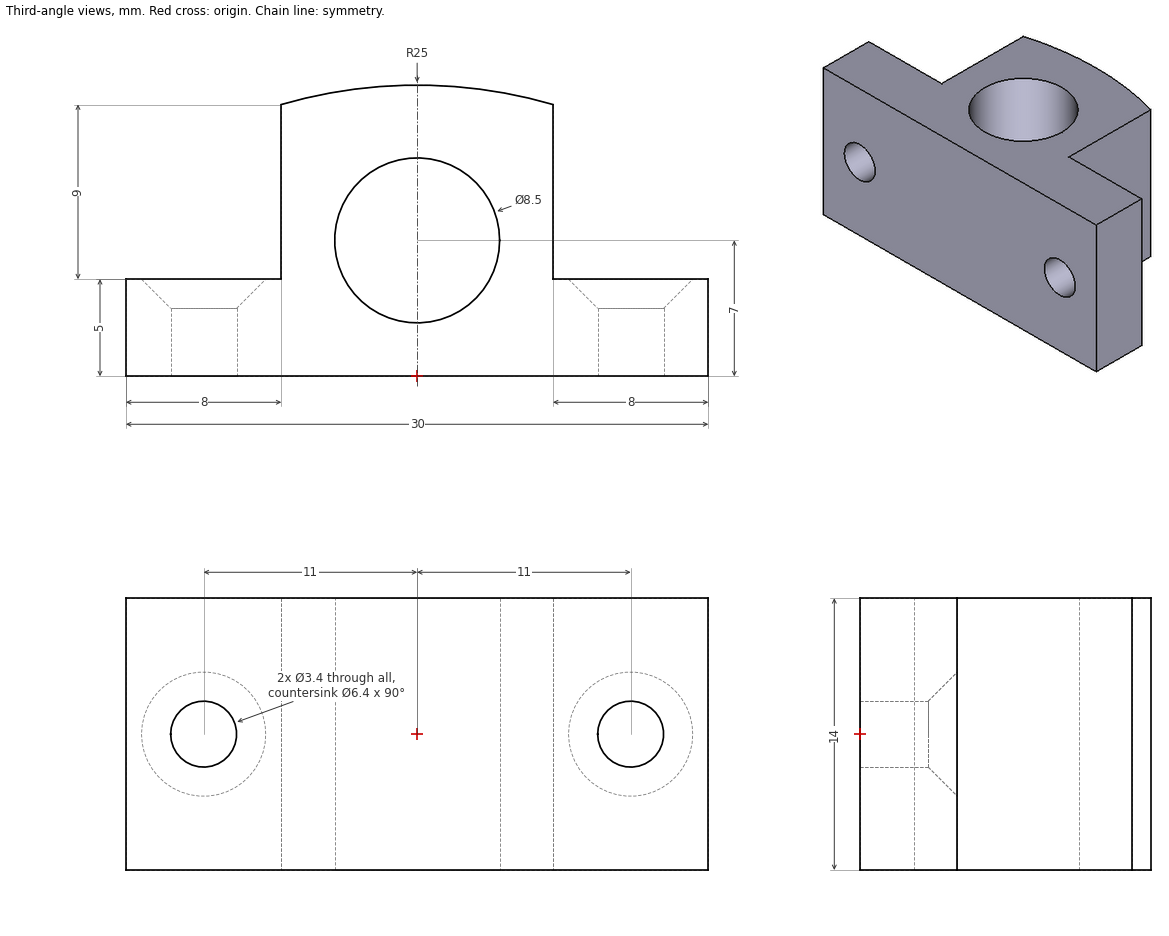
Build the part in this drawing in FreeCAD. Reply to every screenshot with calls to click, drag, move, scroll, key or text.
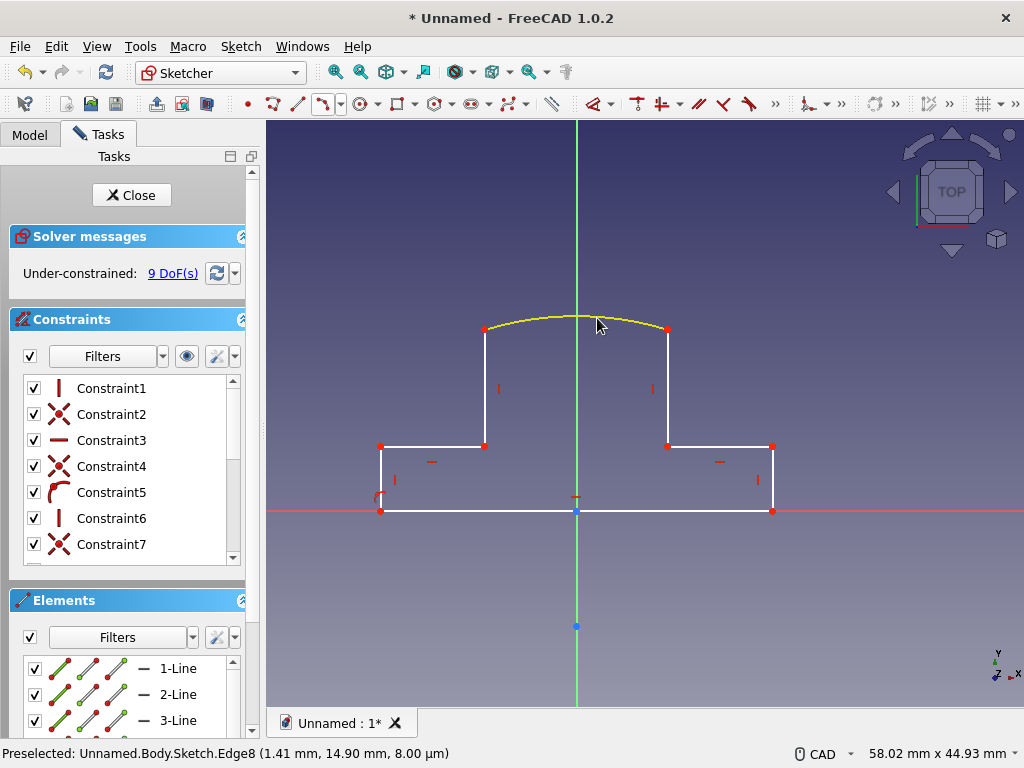
click(576, 627)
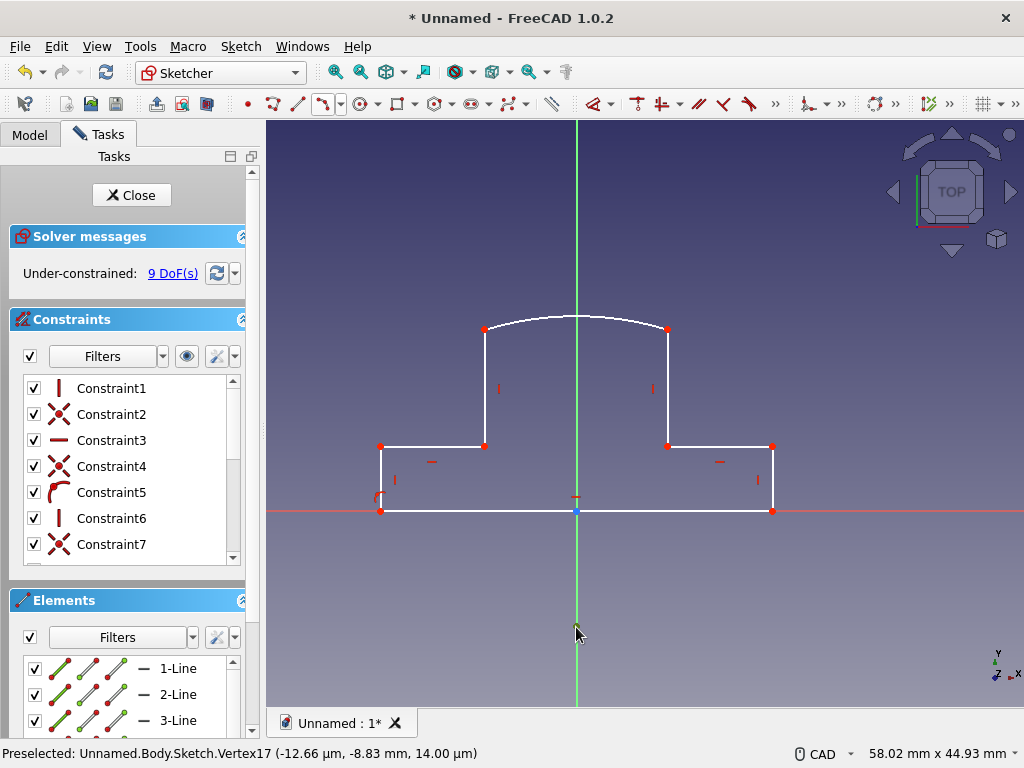
click(577, 641)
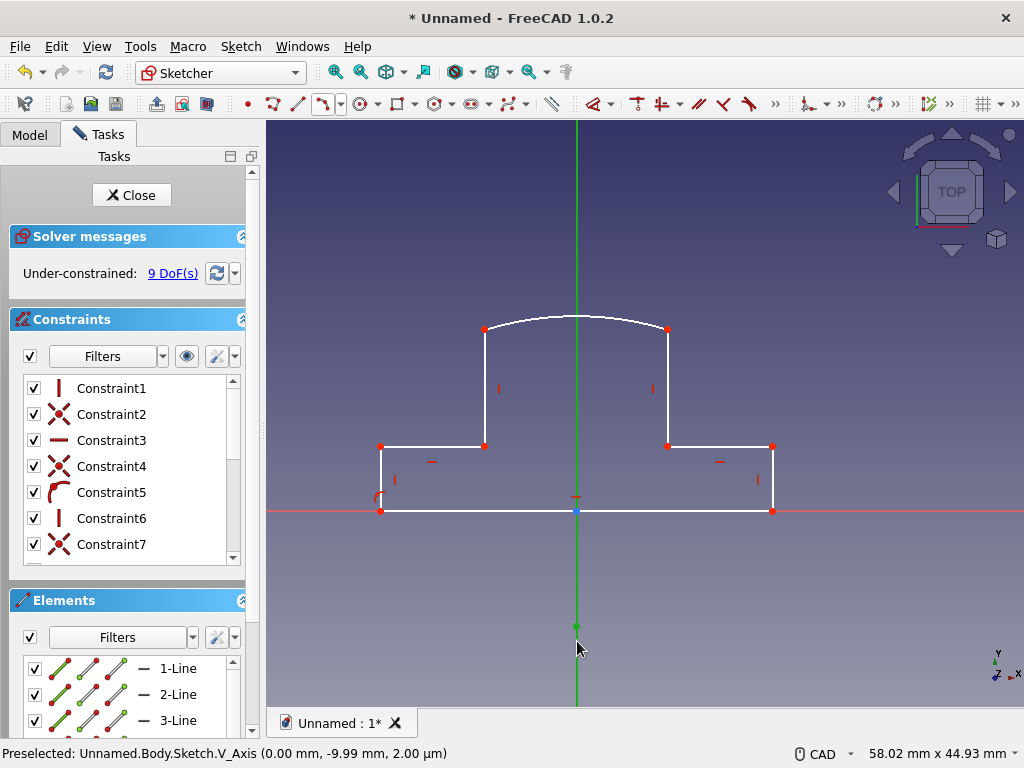
click(637, 104)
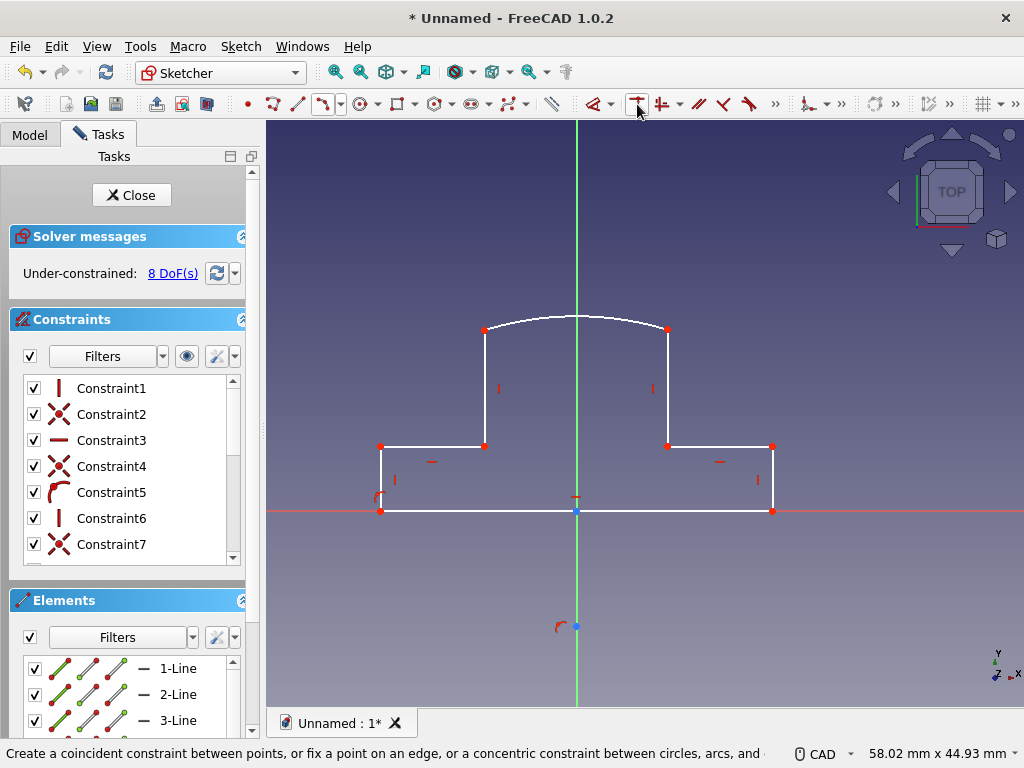
click(381, 447)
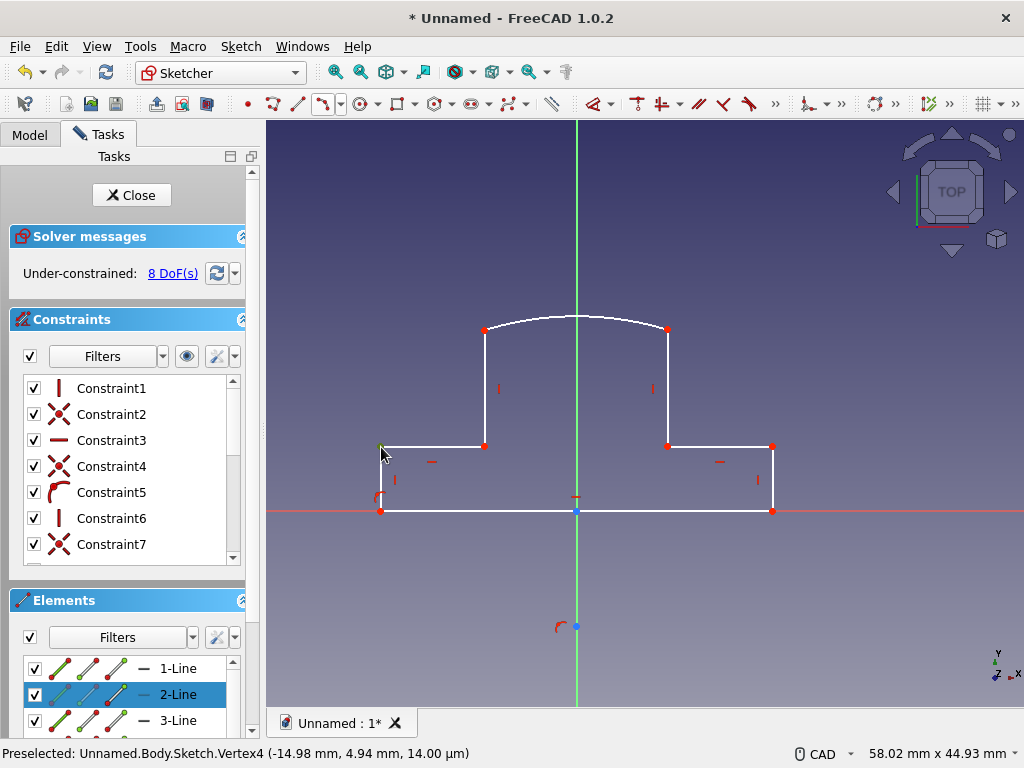
click(773, 447)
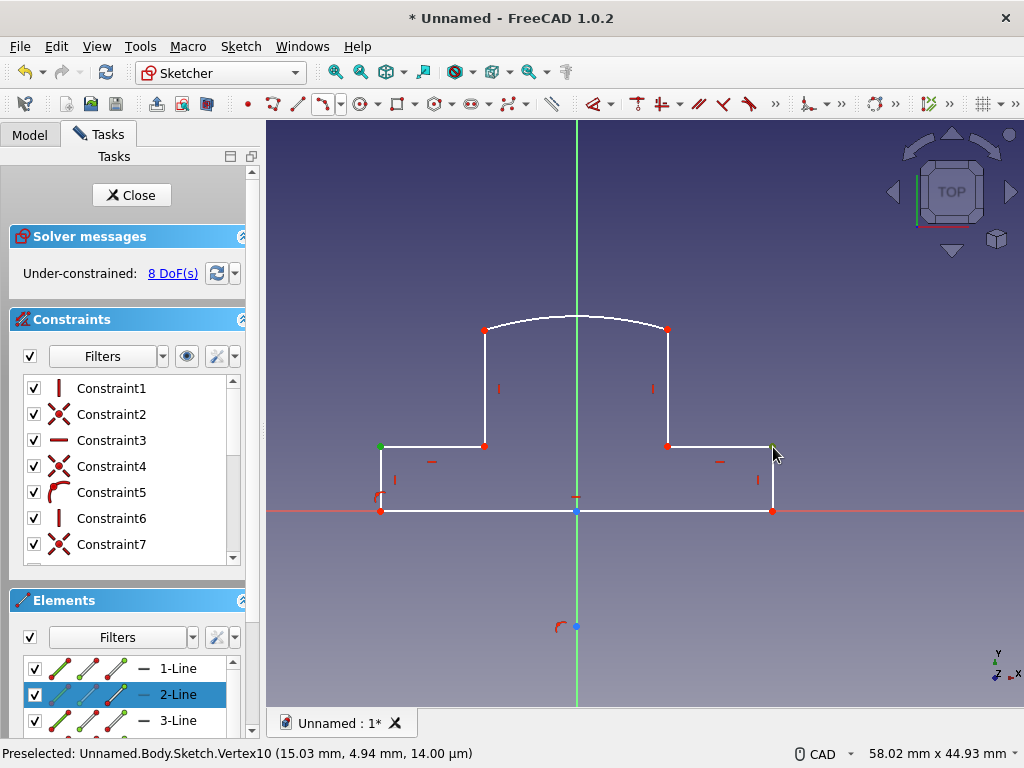
click(577, 641)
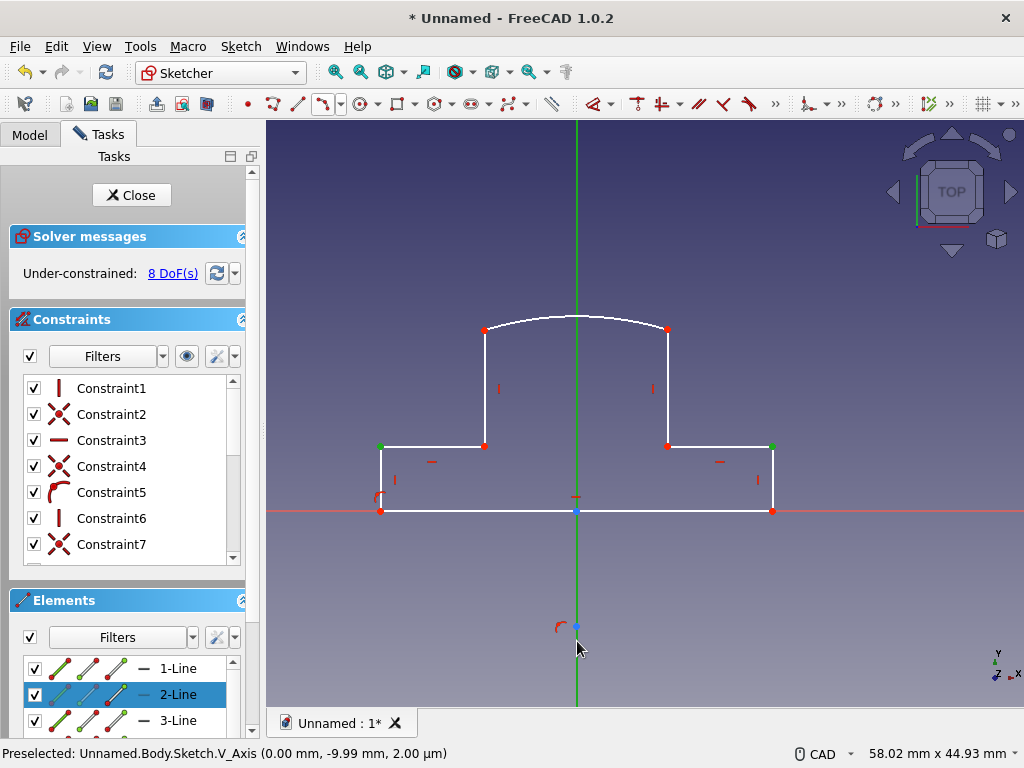
key(s)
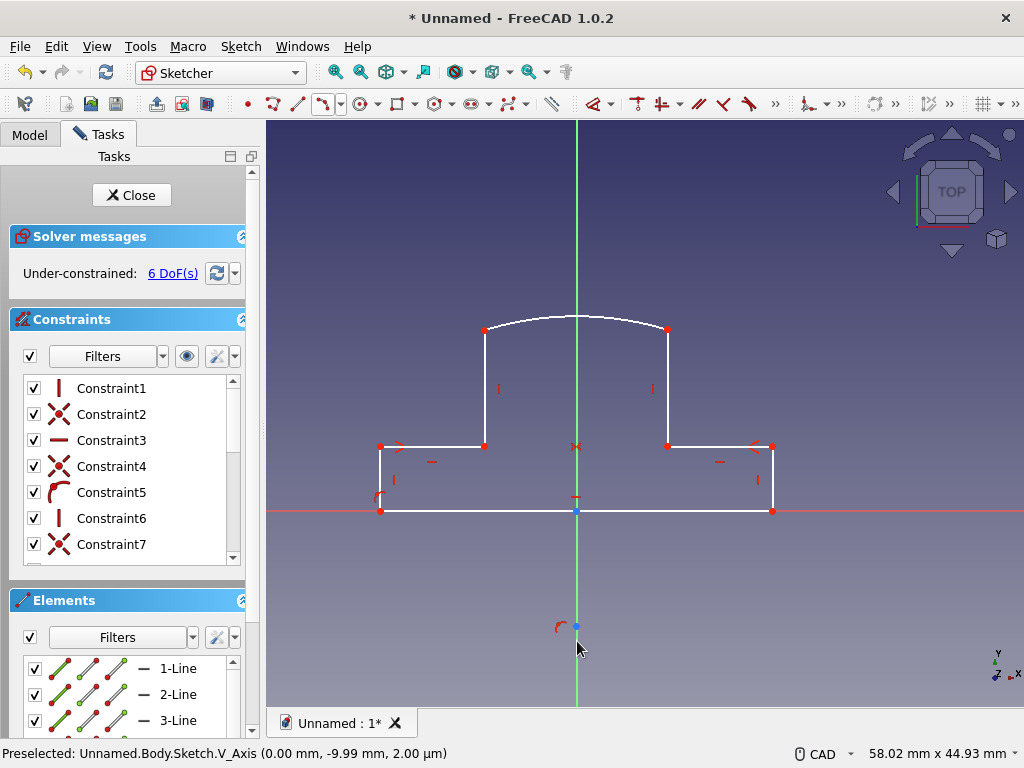
click(592, 104)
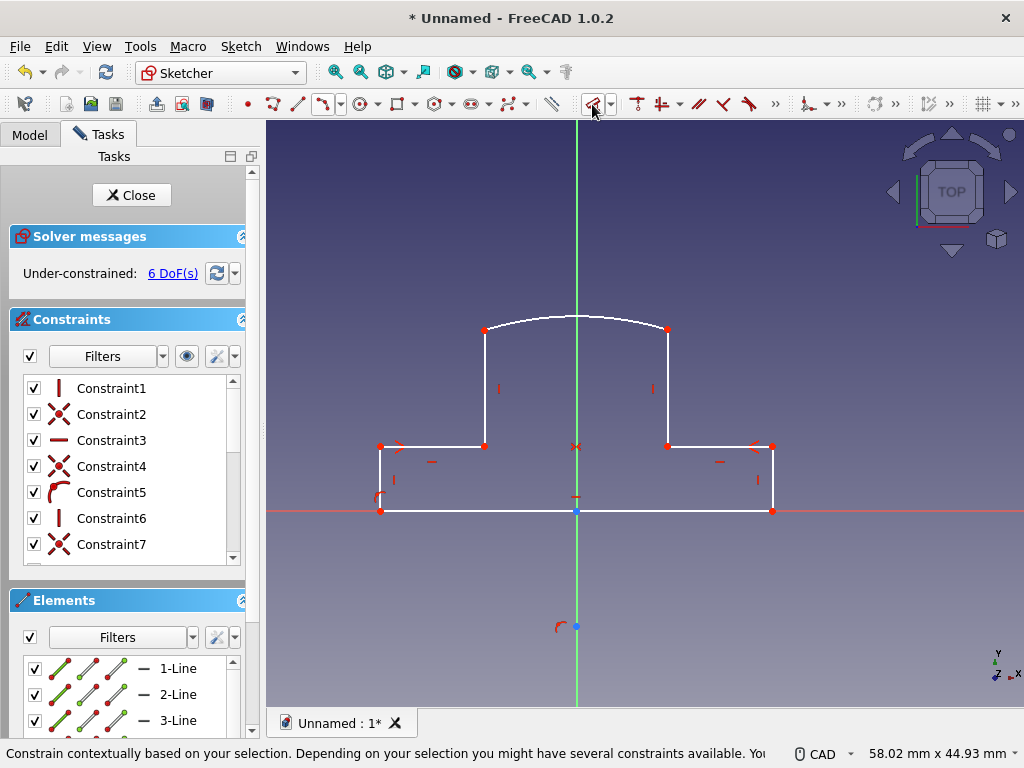
click(614, 318)
click(618, 286)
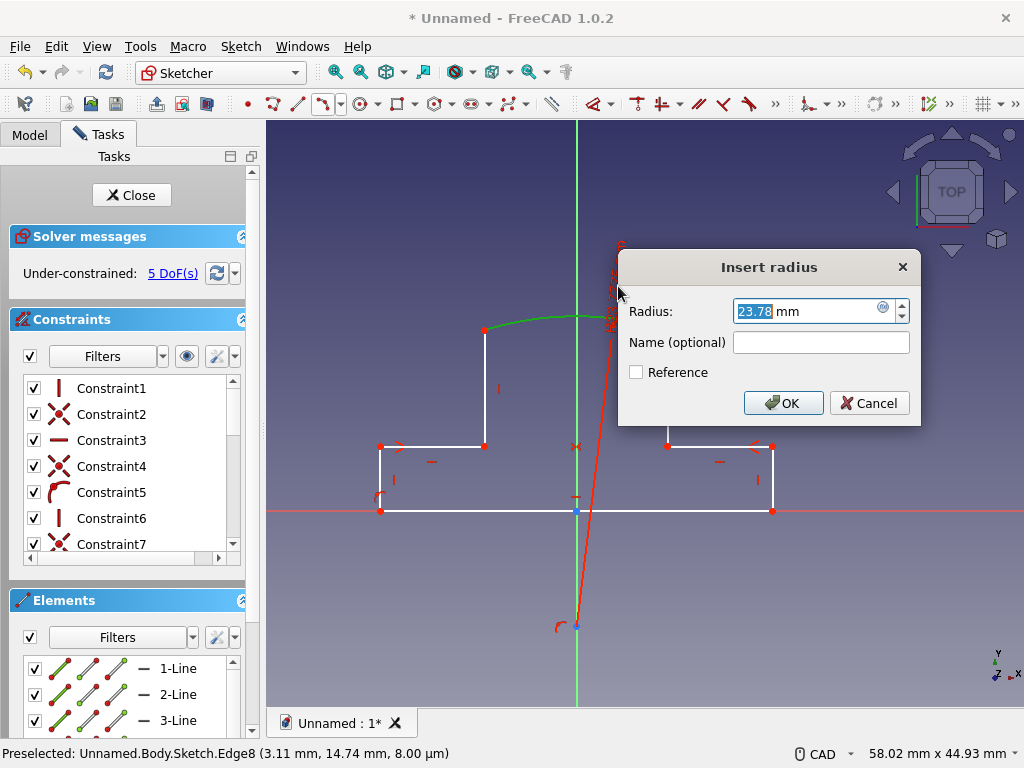
text(25)
key(Return)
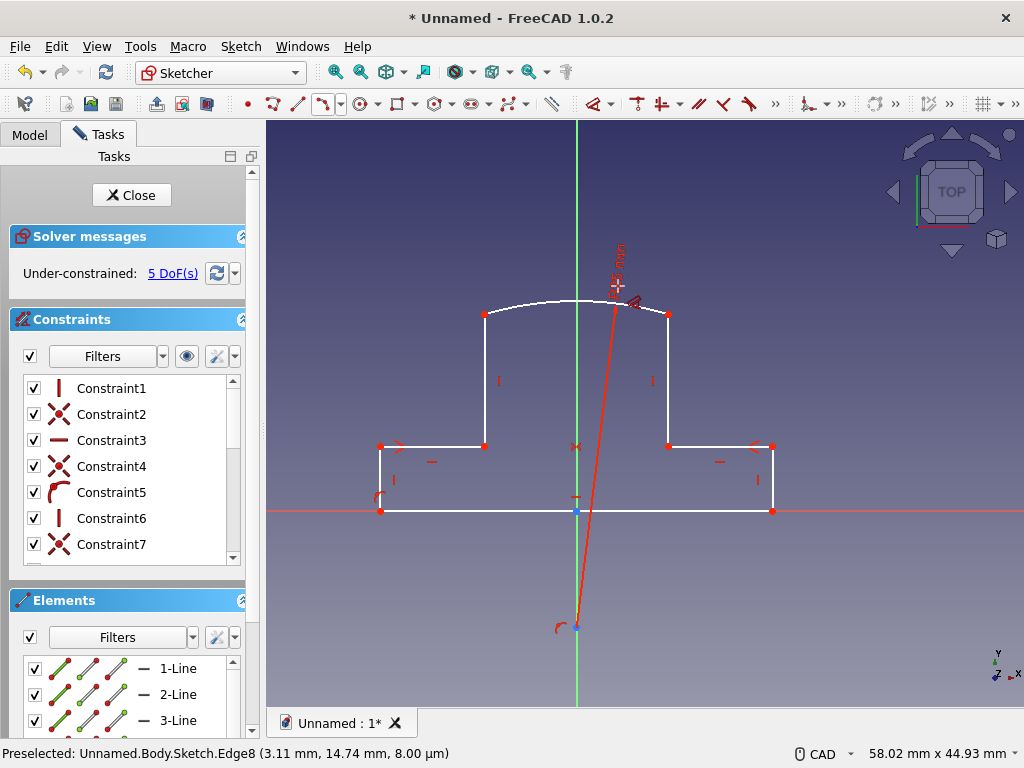
click(485, 354)
click(451, 381)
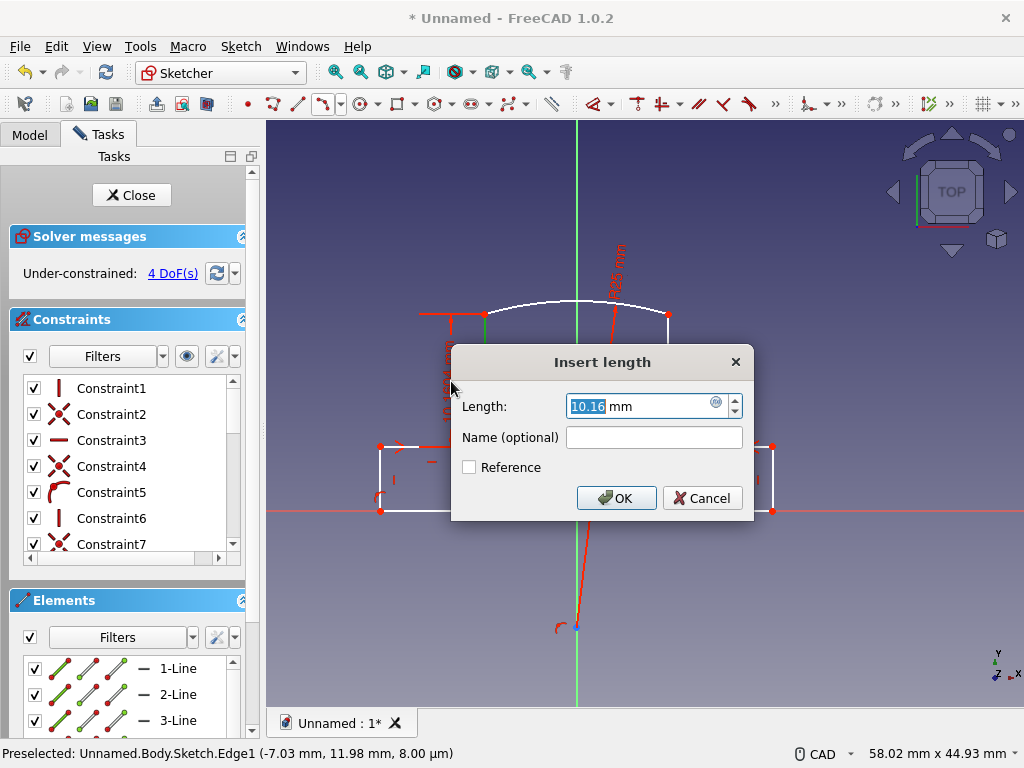
text(9)
key(Return)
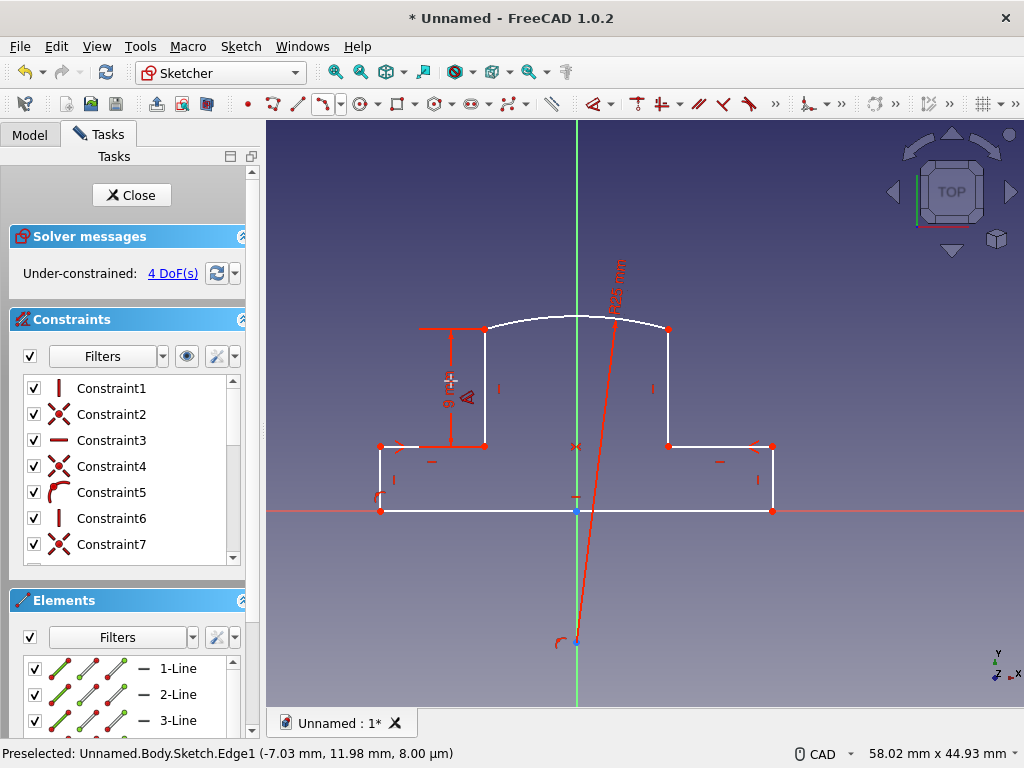
click(454, 447)
click(433, 481)